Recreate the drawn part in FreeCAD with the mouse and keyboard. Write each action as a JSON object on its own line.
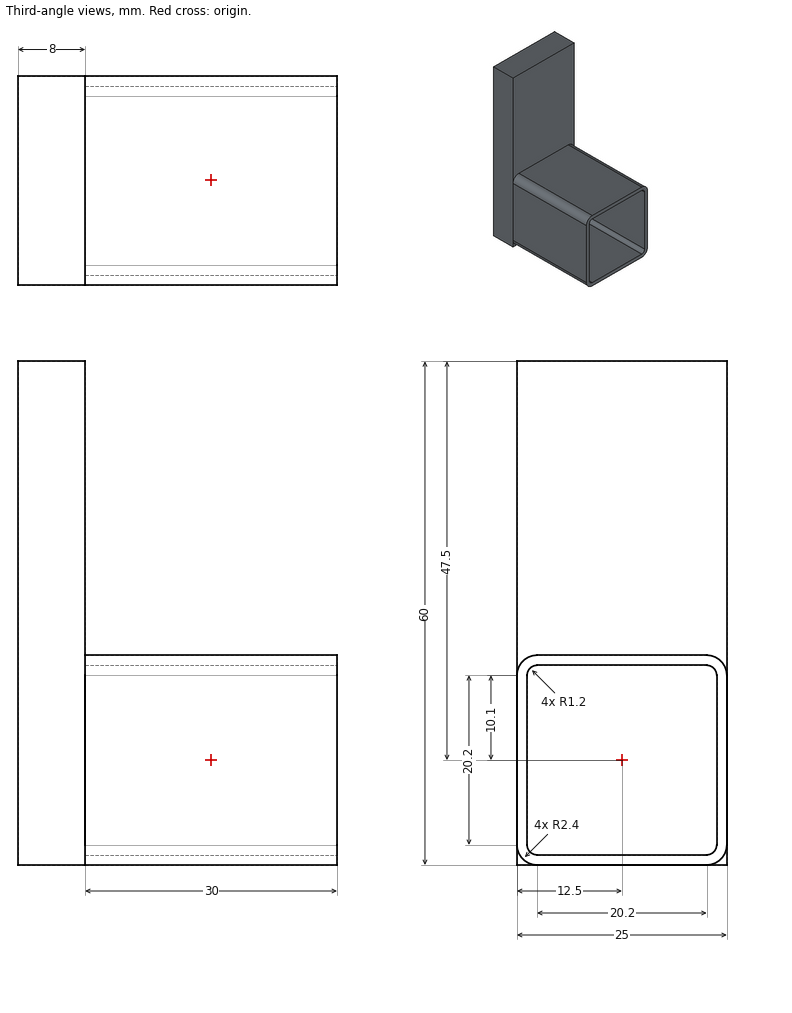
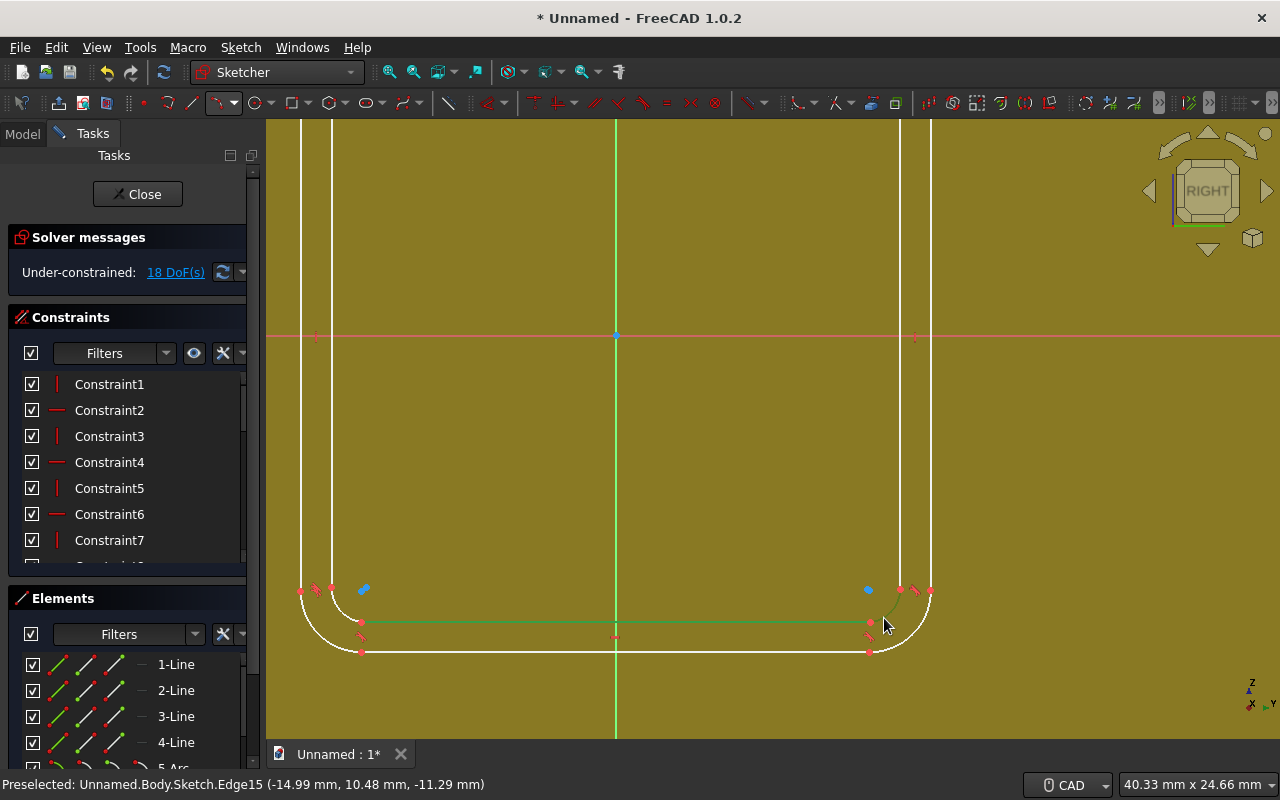
{"action": "key", "text": "t"}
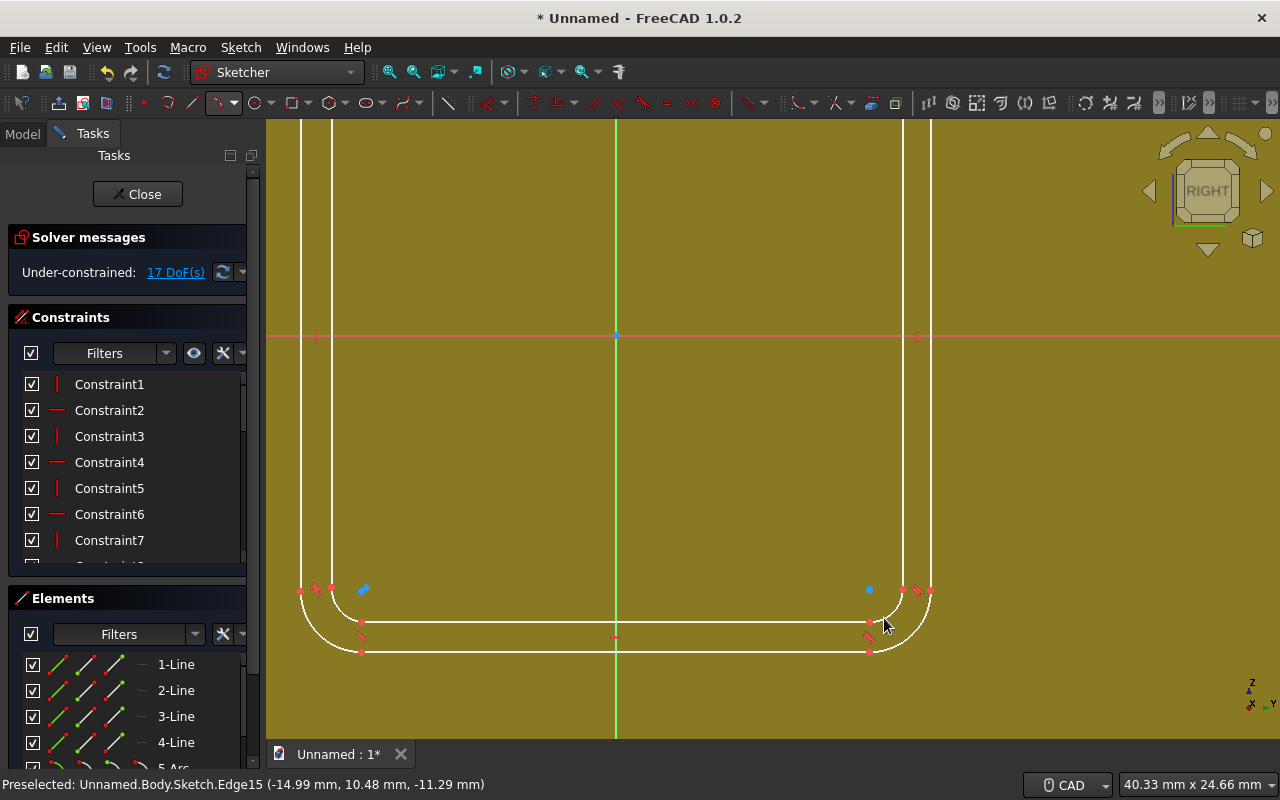
{"action": "left_click", "coordinate": [717, 622]}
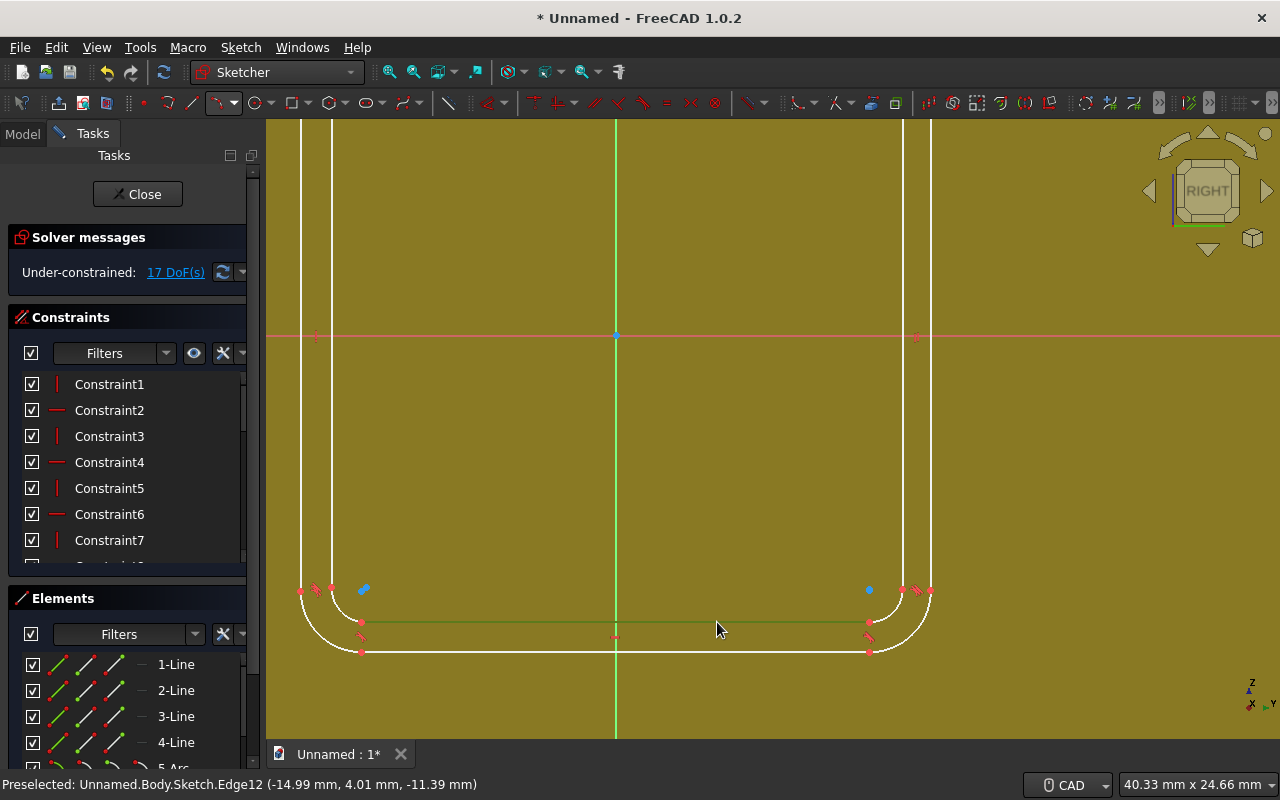
{"action": "left_click", "coordinate": [335, 602]}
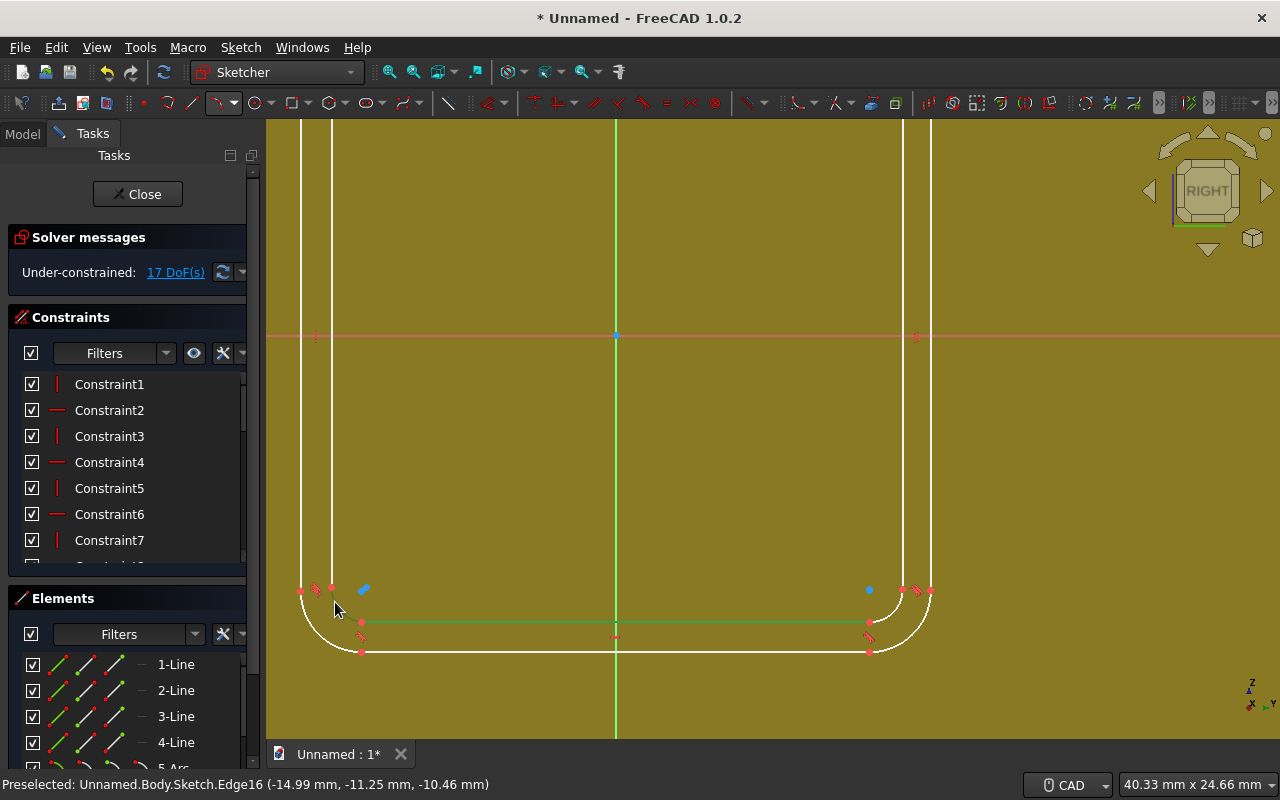
{"action": "key", "text": "t"}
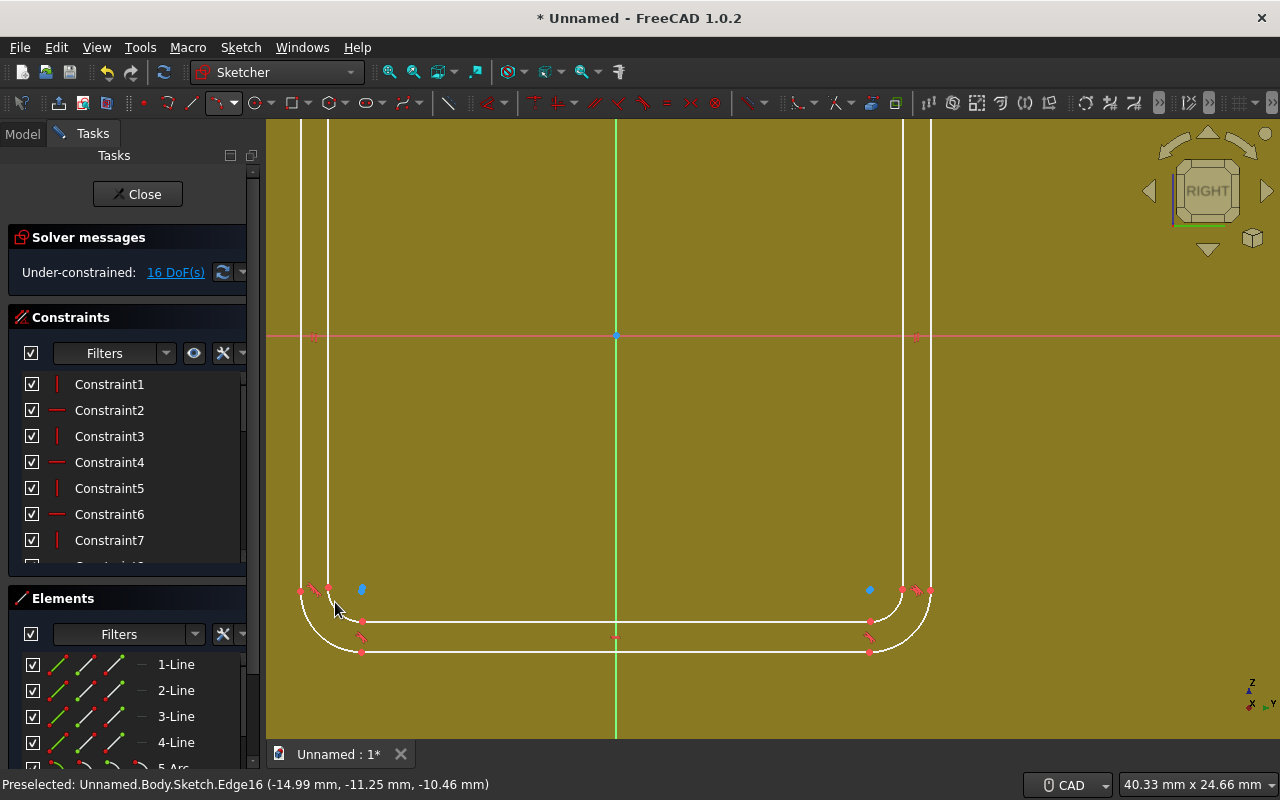
{"action": "scroll", "coordinate": [884, 618], "scroll_direction": "down", "scroll_amount": 2}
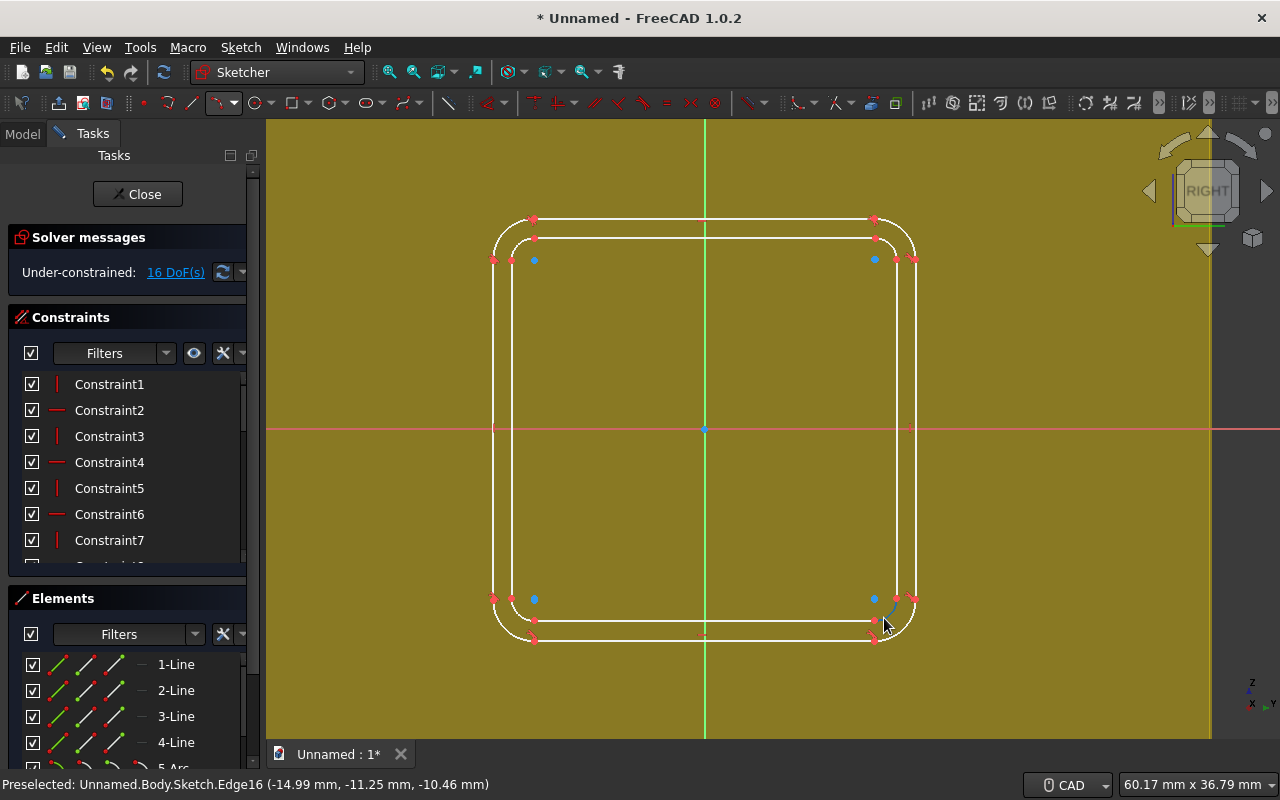
{"action": "left_click", "coordinate": [516, 223]}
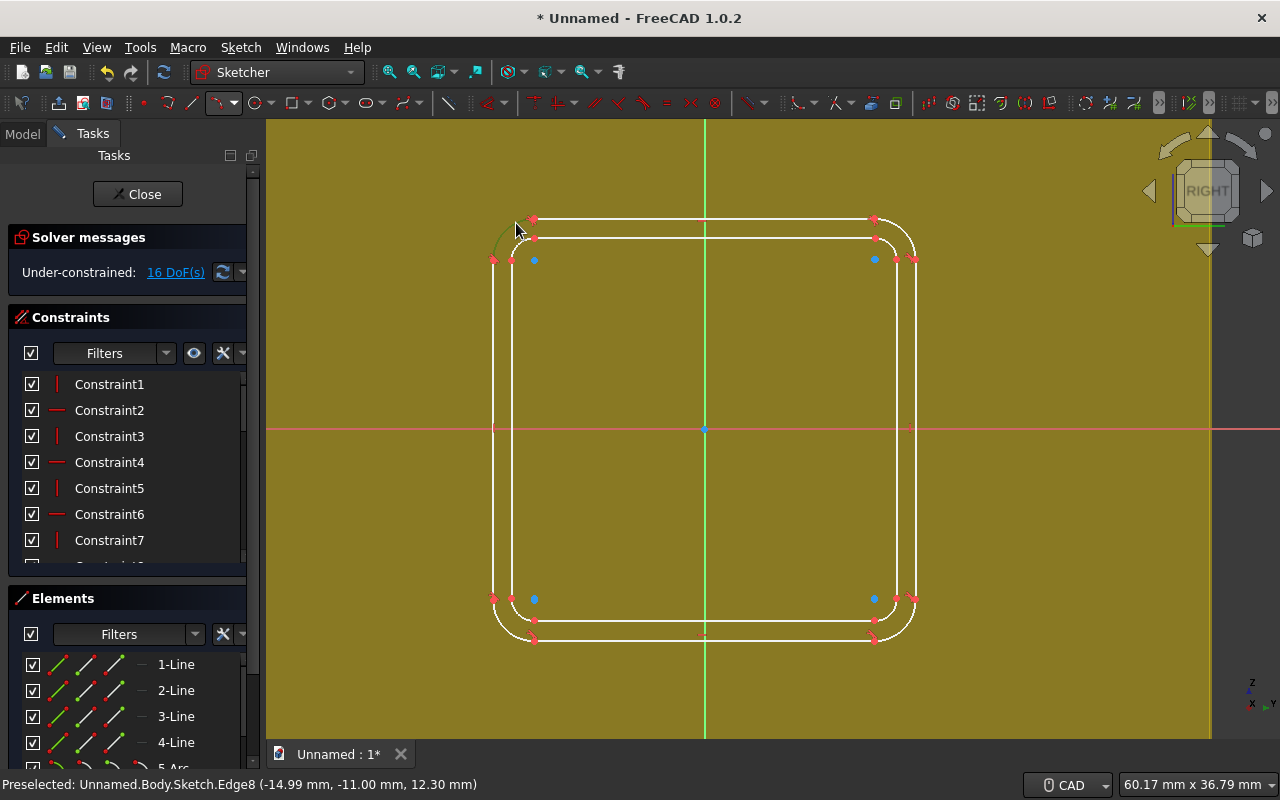
{"action": "scroll", "coordinate": [524, 241], "scroll_direction": "up", "scroll_amount": 2}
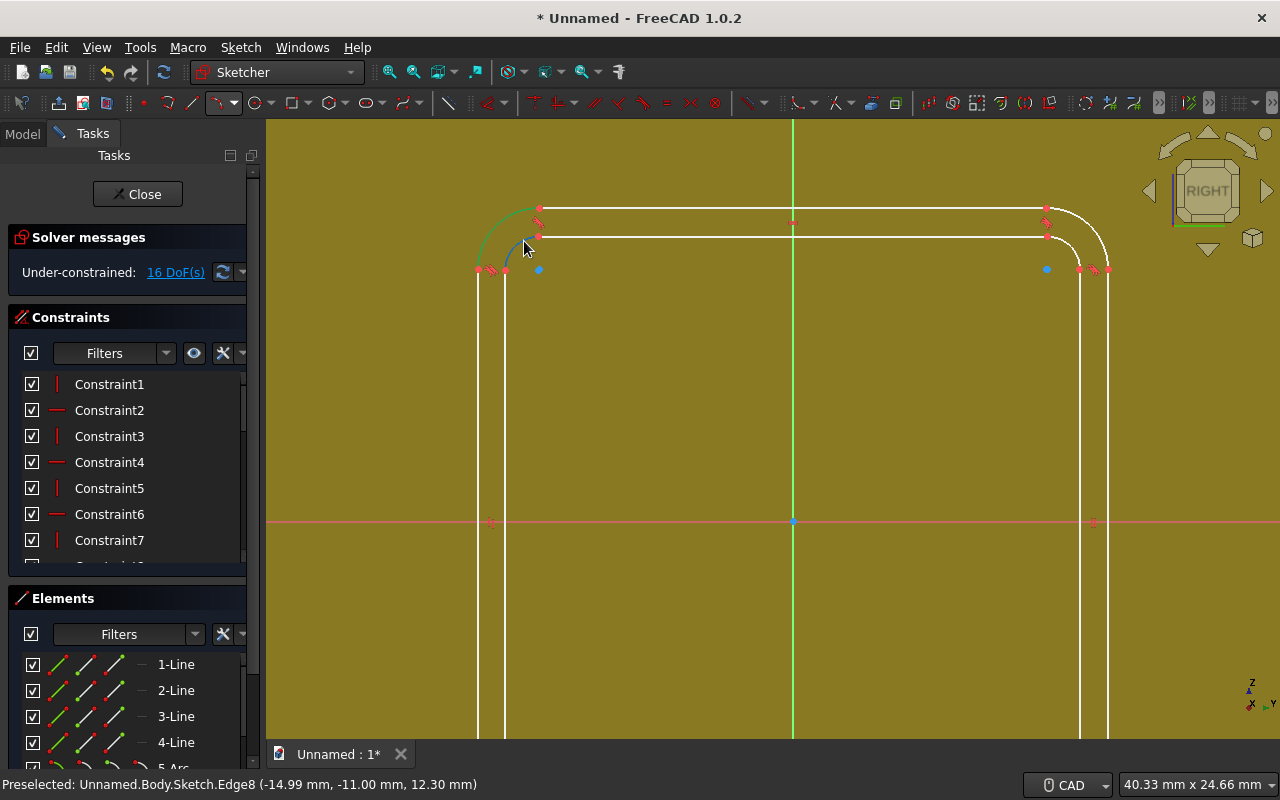
{"action": "left_click", "coordinate": [524, 240]}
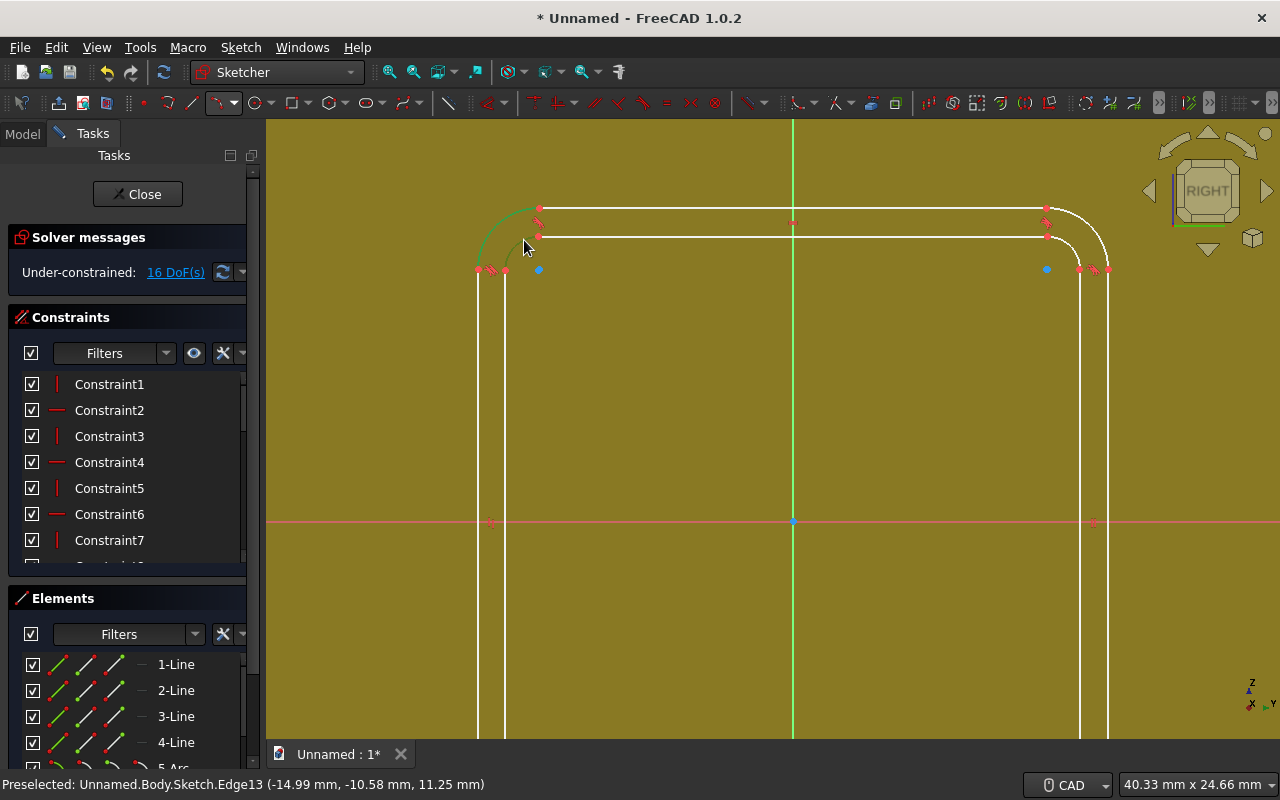
{"action": "key", "text": "c"}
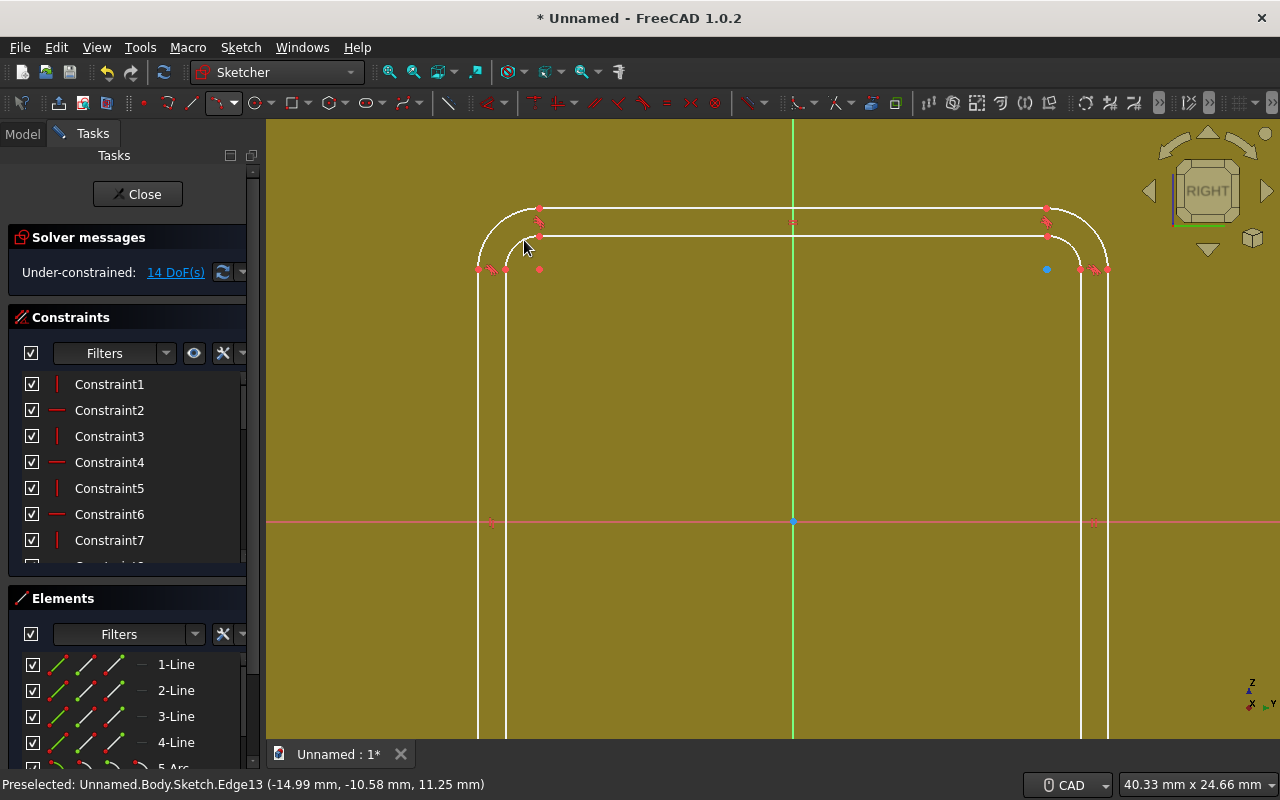
{"action": "left_click", "coordinate": [1101, 242]}